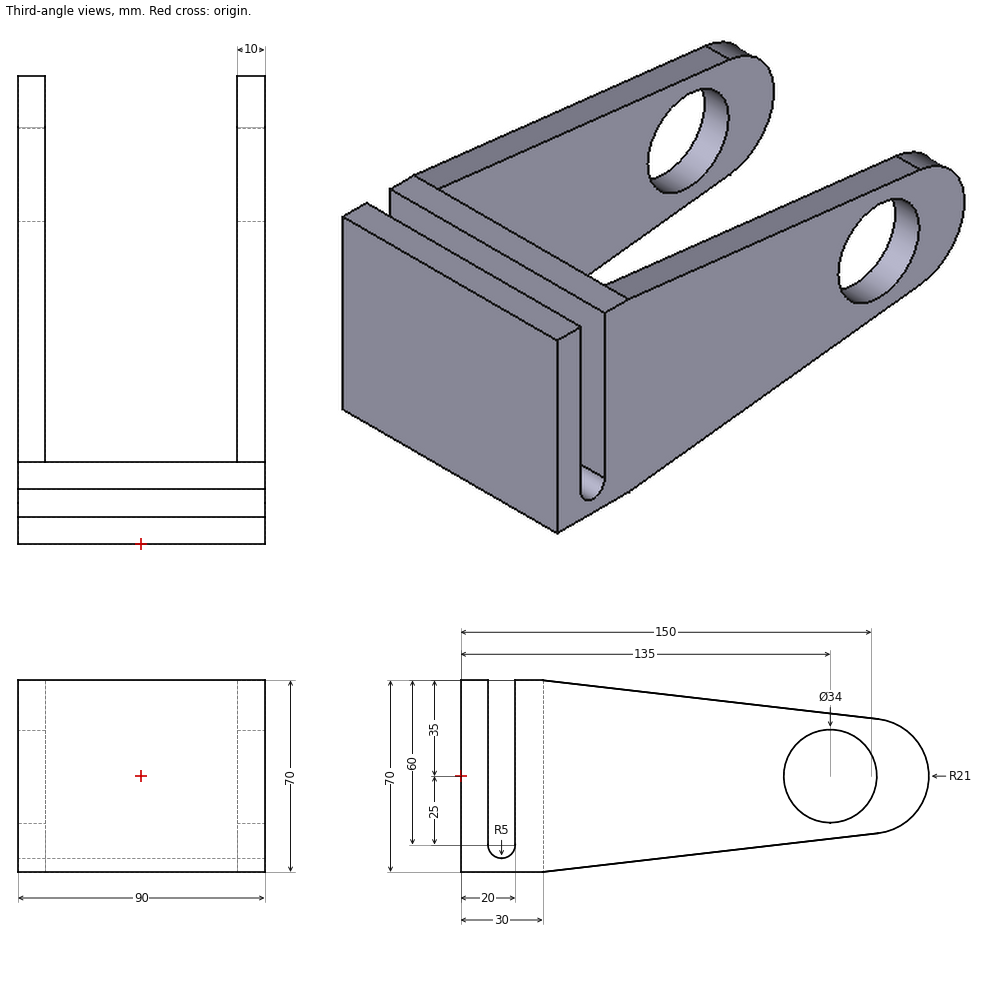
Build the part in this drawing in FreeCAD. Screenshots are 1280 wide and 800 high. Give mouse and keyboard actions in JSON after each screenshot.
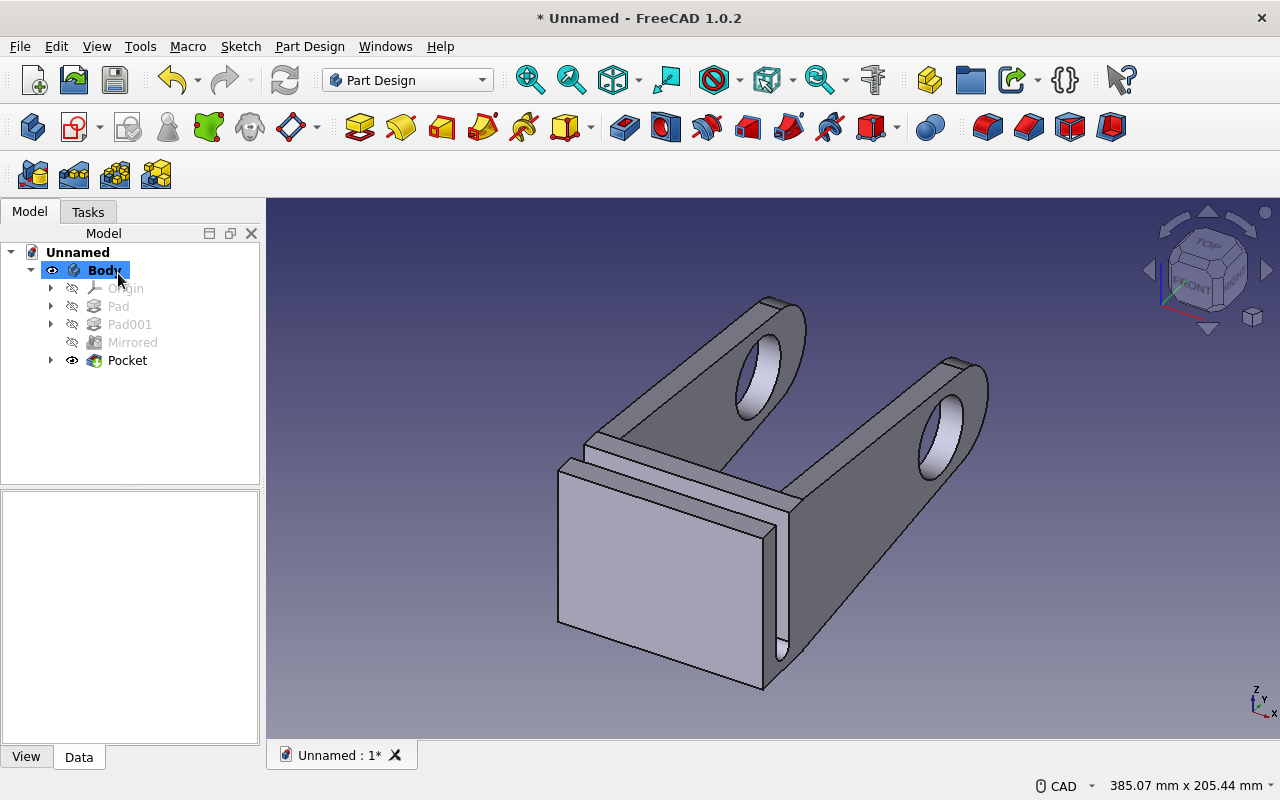
{"action": "key", "text": "0"}